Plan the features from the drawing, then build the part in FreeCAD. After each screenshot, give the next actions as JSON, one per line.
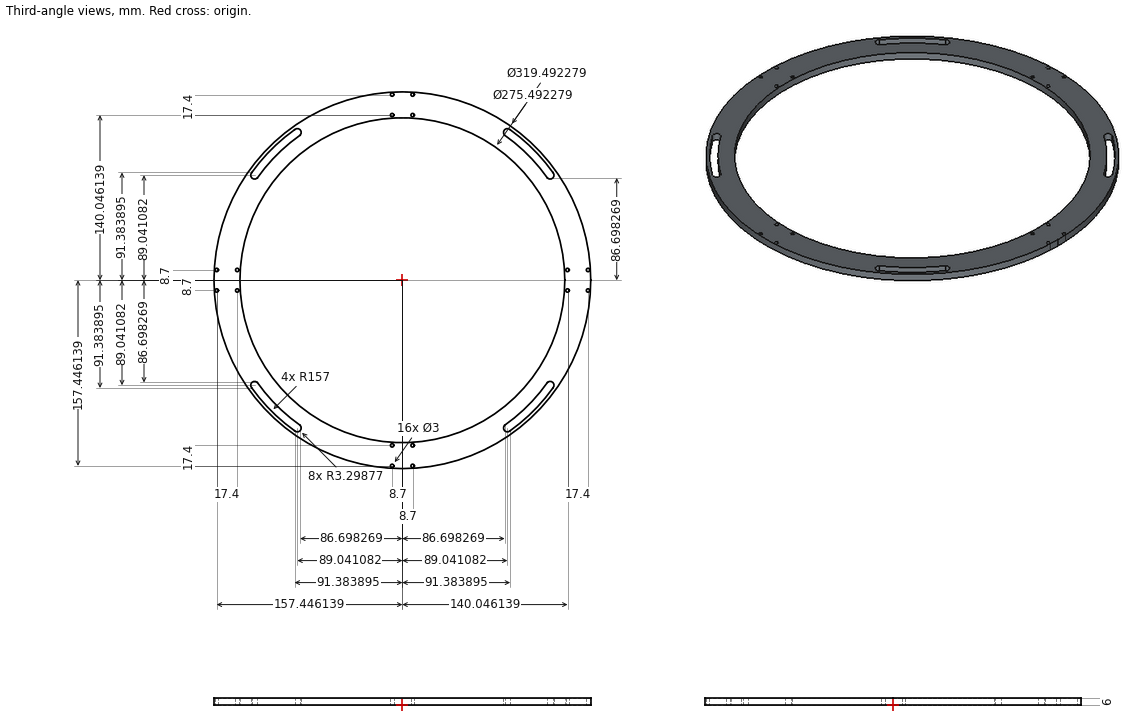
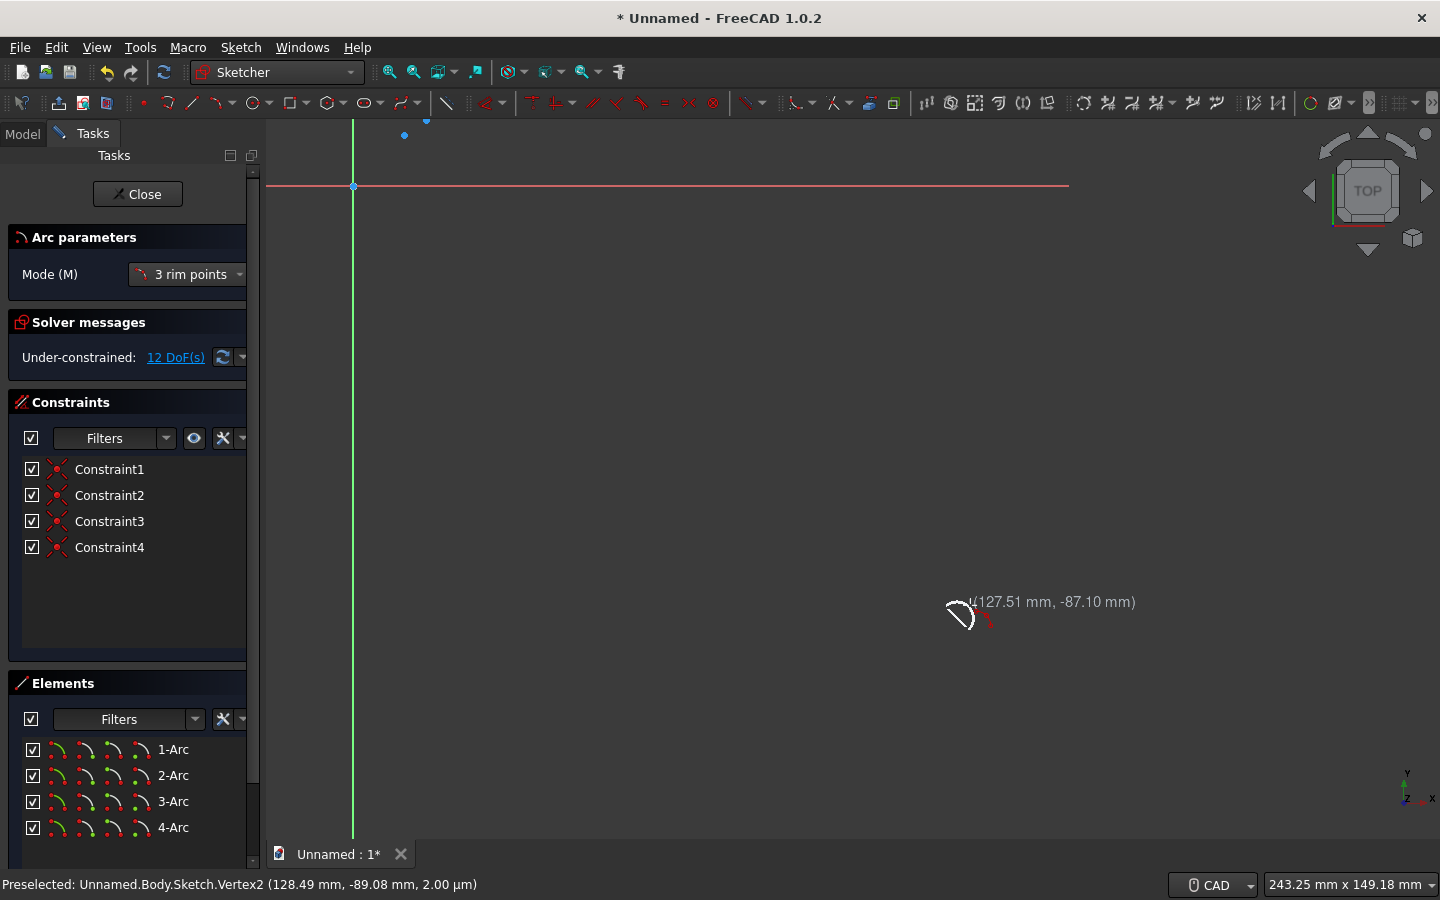
{"action": "left_click", "coordinate": [969, 605]}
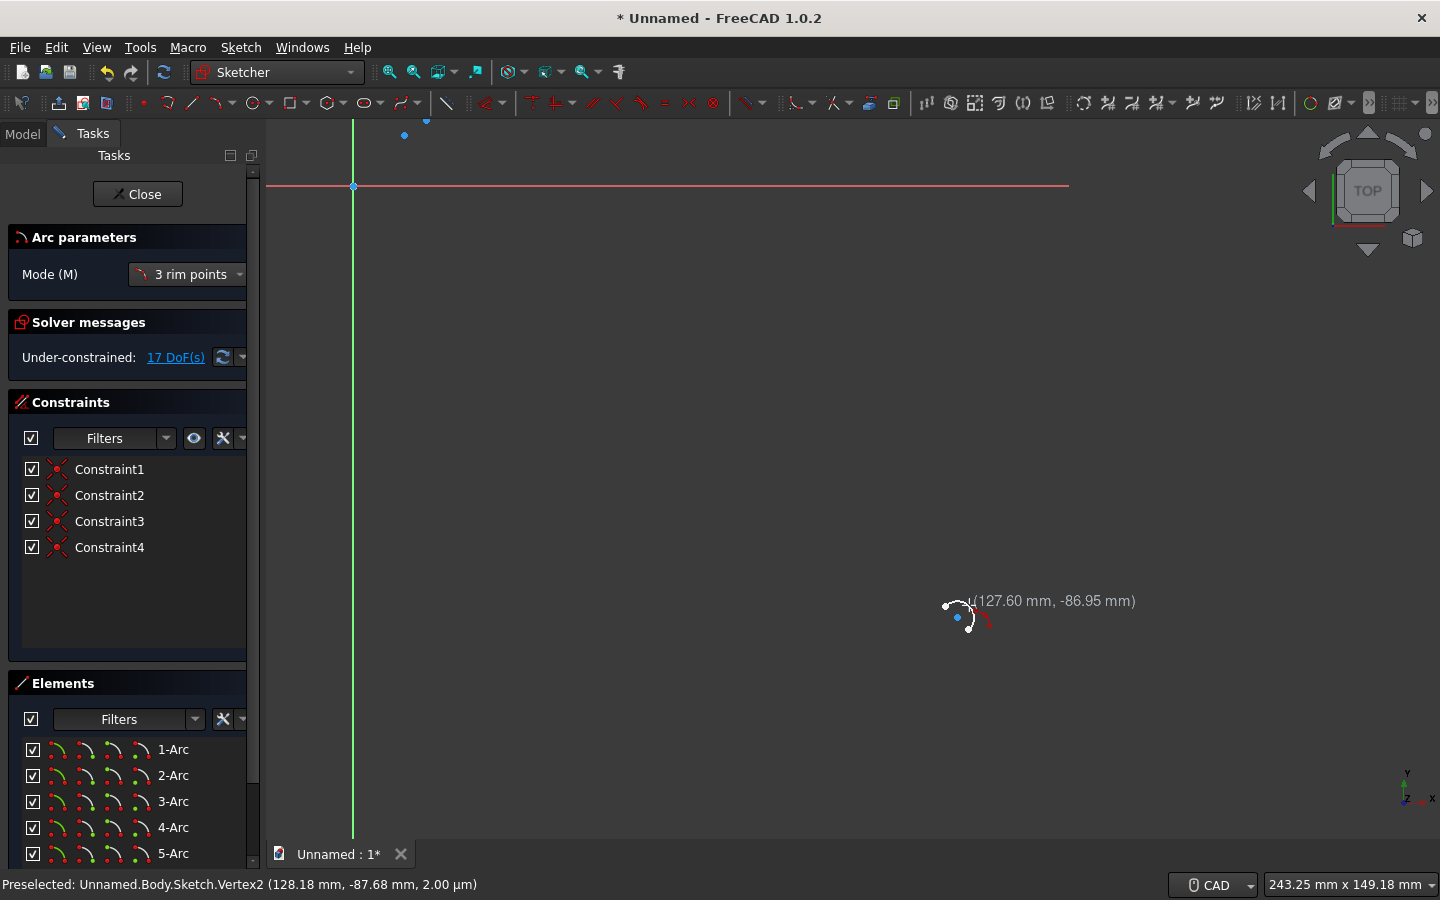
{"action": "left_click", "coordinate": [969, 630]}
{"action": "left_click", "coordinate": [794, 803]}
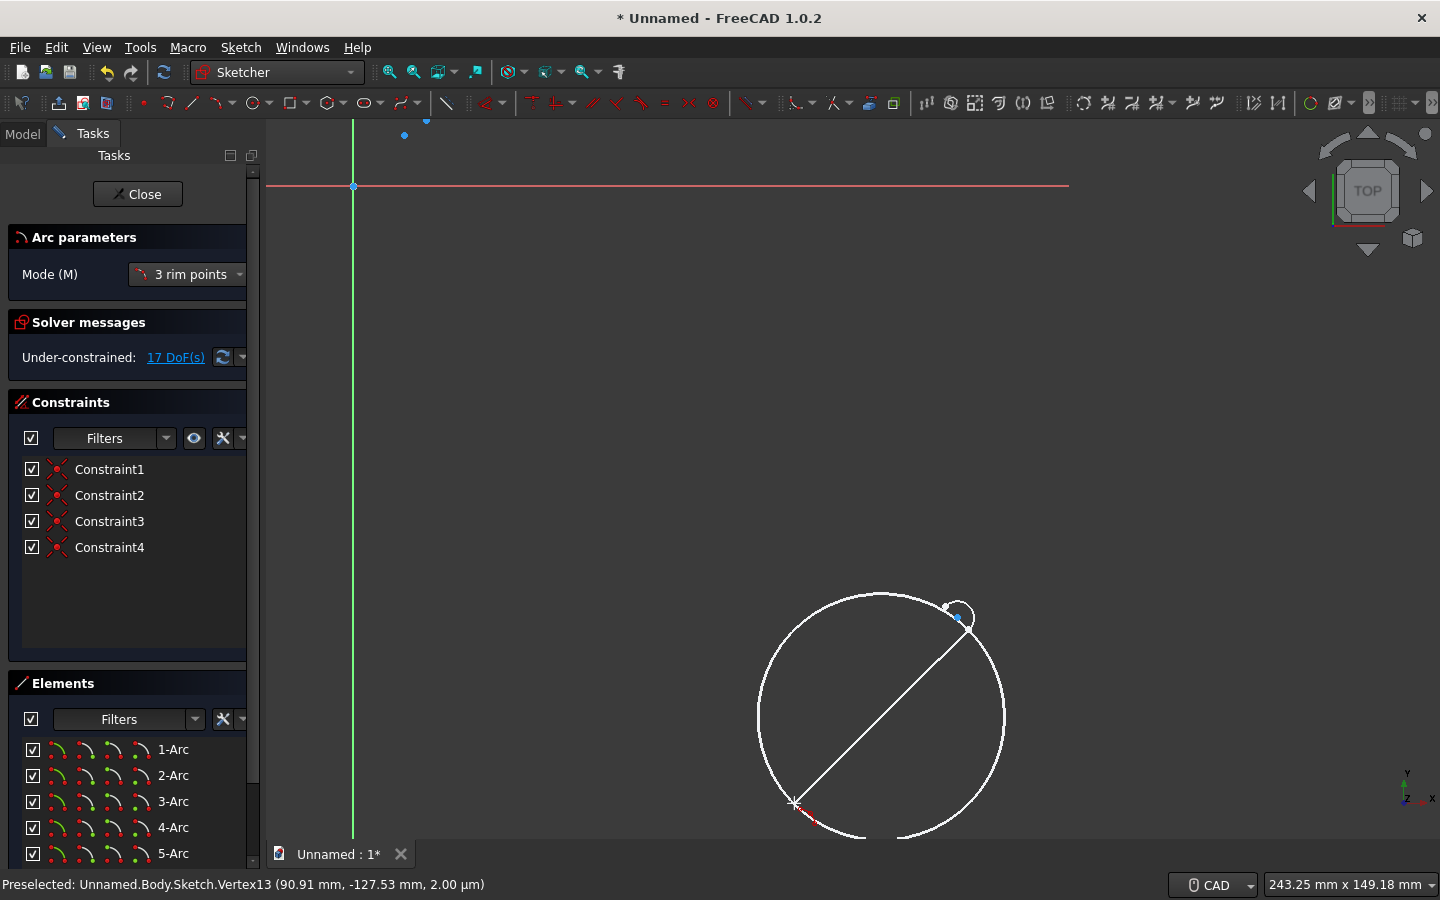
{"action": "scroll", "coordinate": [889, 722], "scroll_direction": "up", "scroll_amount": 3}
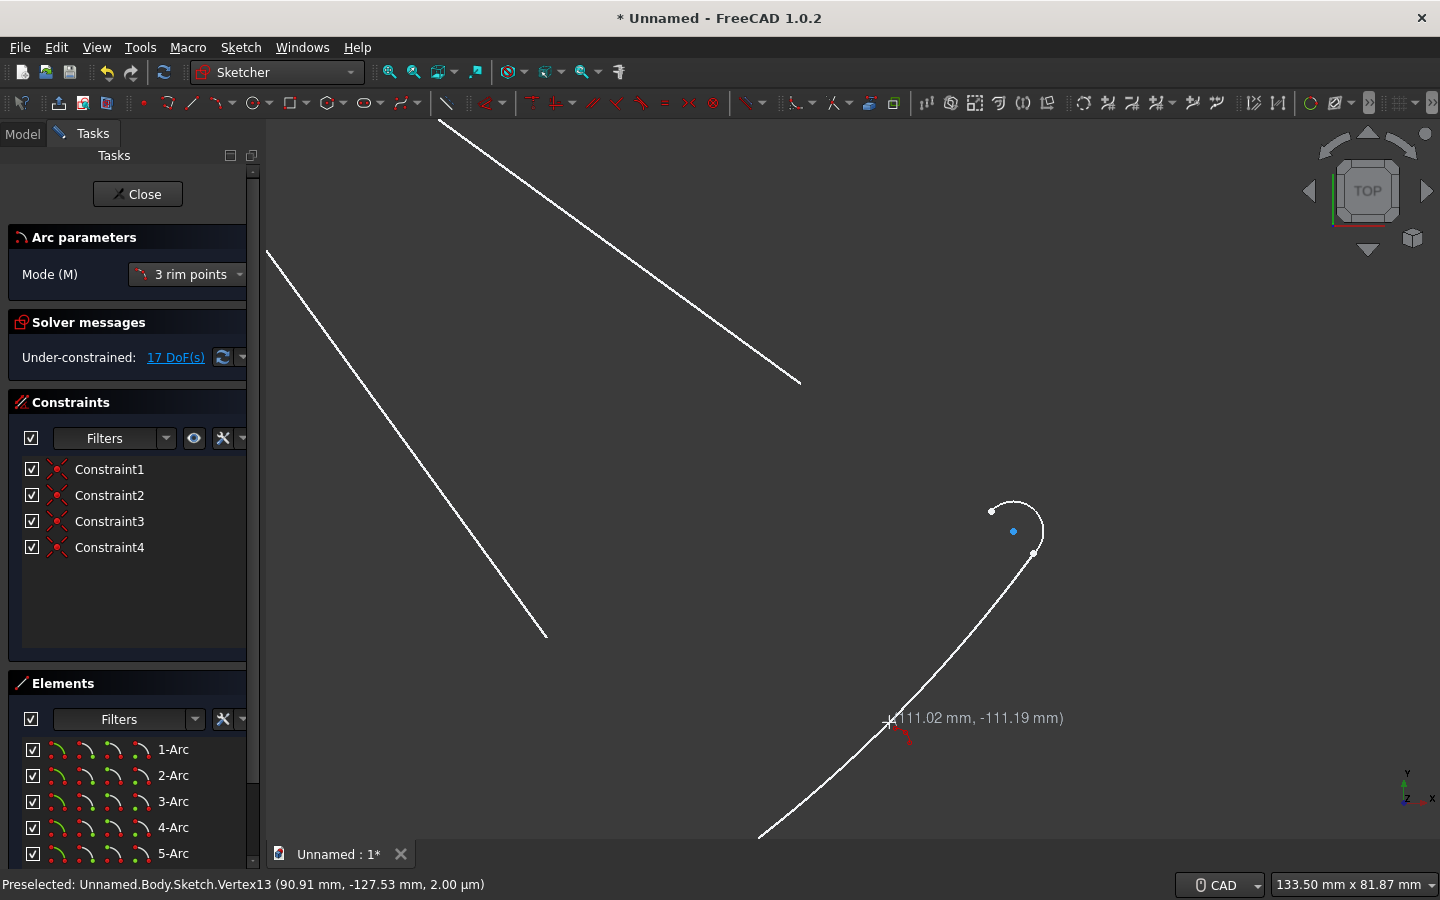
{"action": "left_click", "coordinate": [889, 722]}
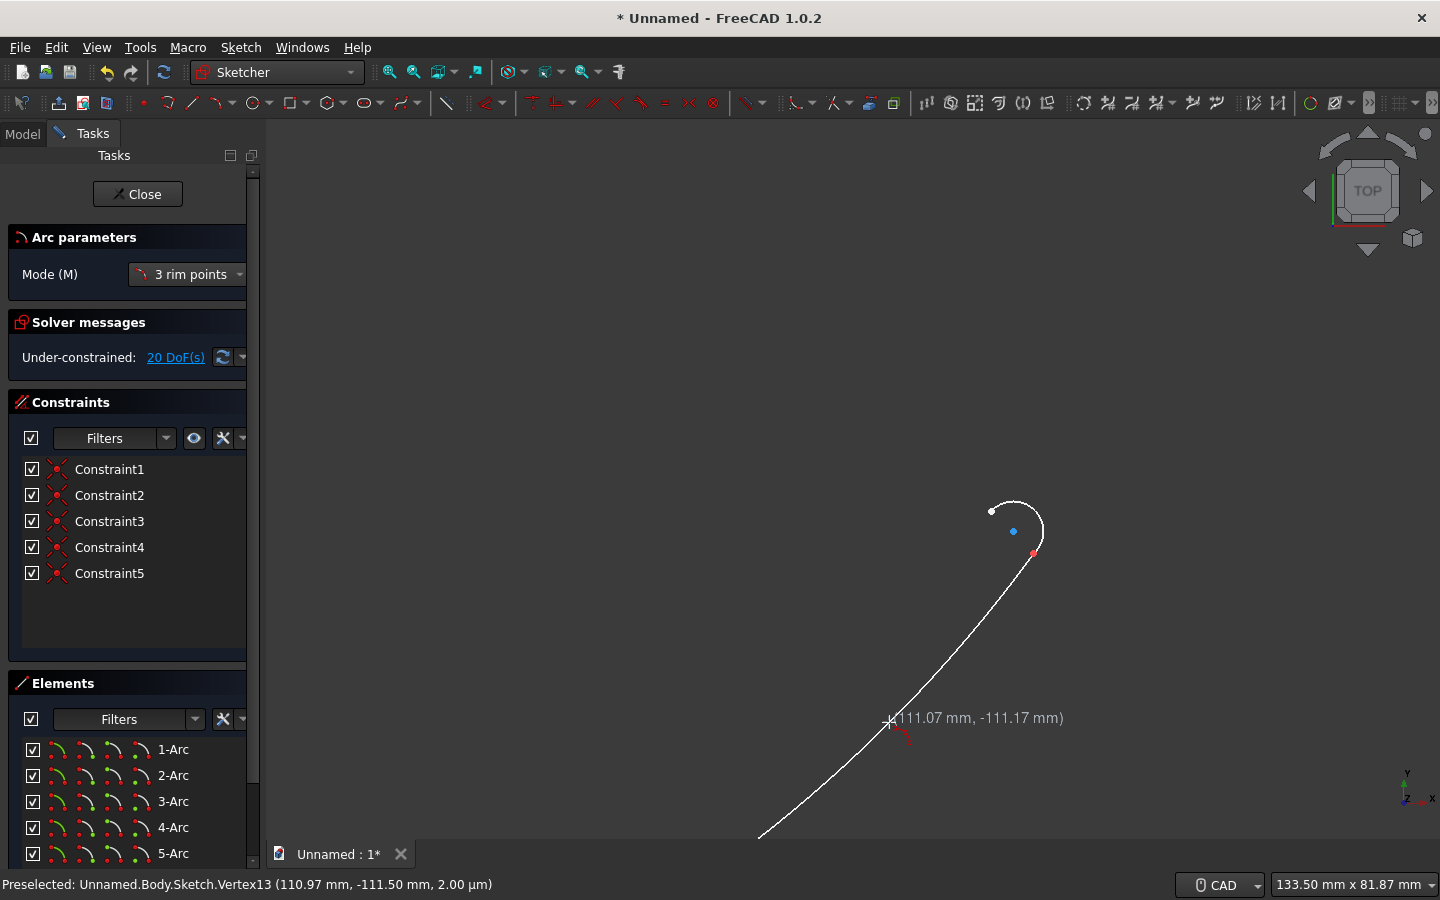
{"action": "scroll", "coordinate": [957, 624], "scroll_direction": "down", "scroll_amount": 9}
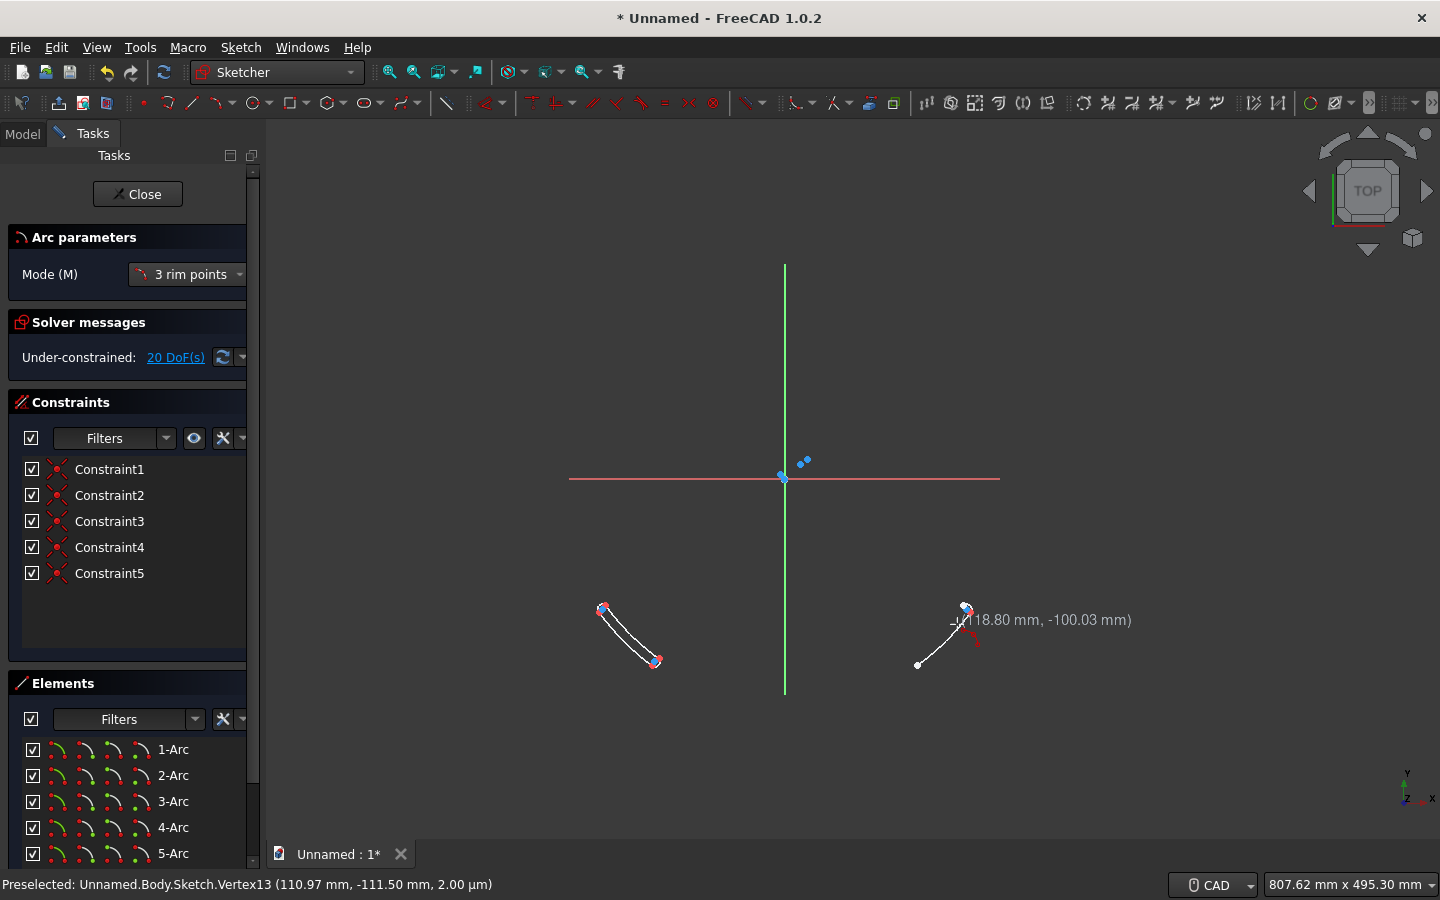
{"action": "left_click", "coordinate": [918, 665]}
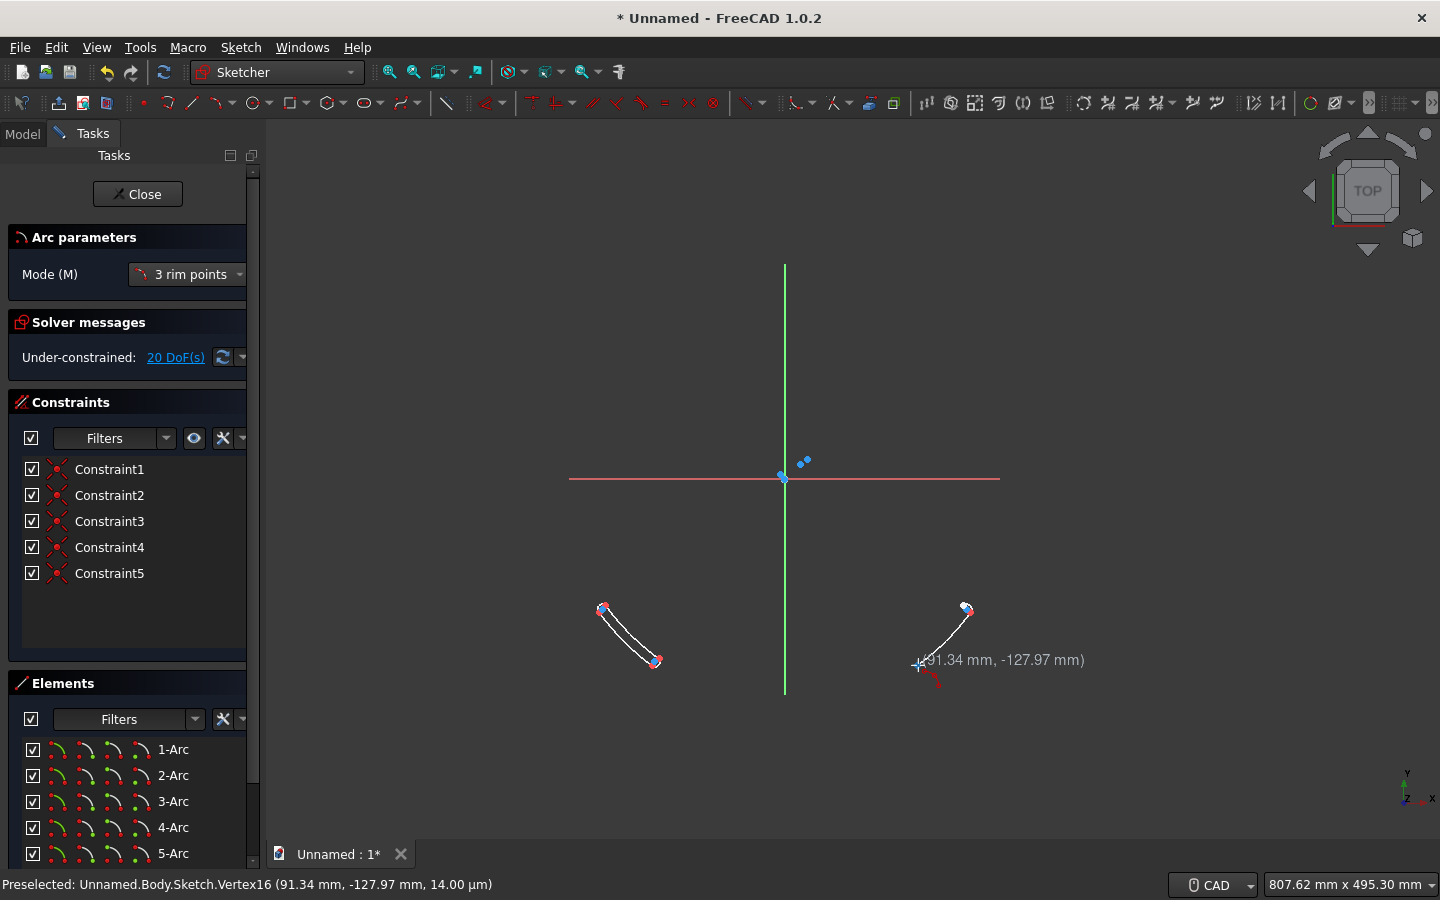
{"action": "scroll", "coordinate": [911, 658], "scroll_direction": "up", "scroll_amount": 3}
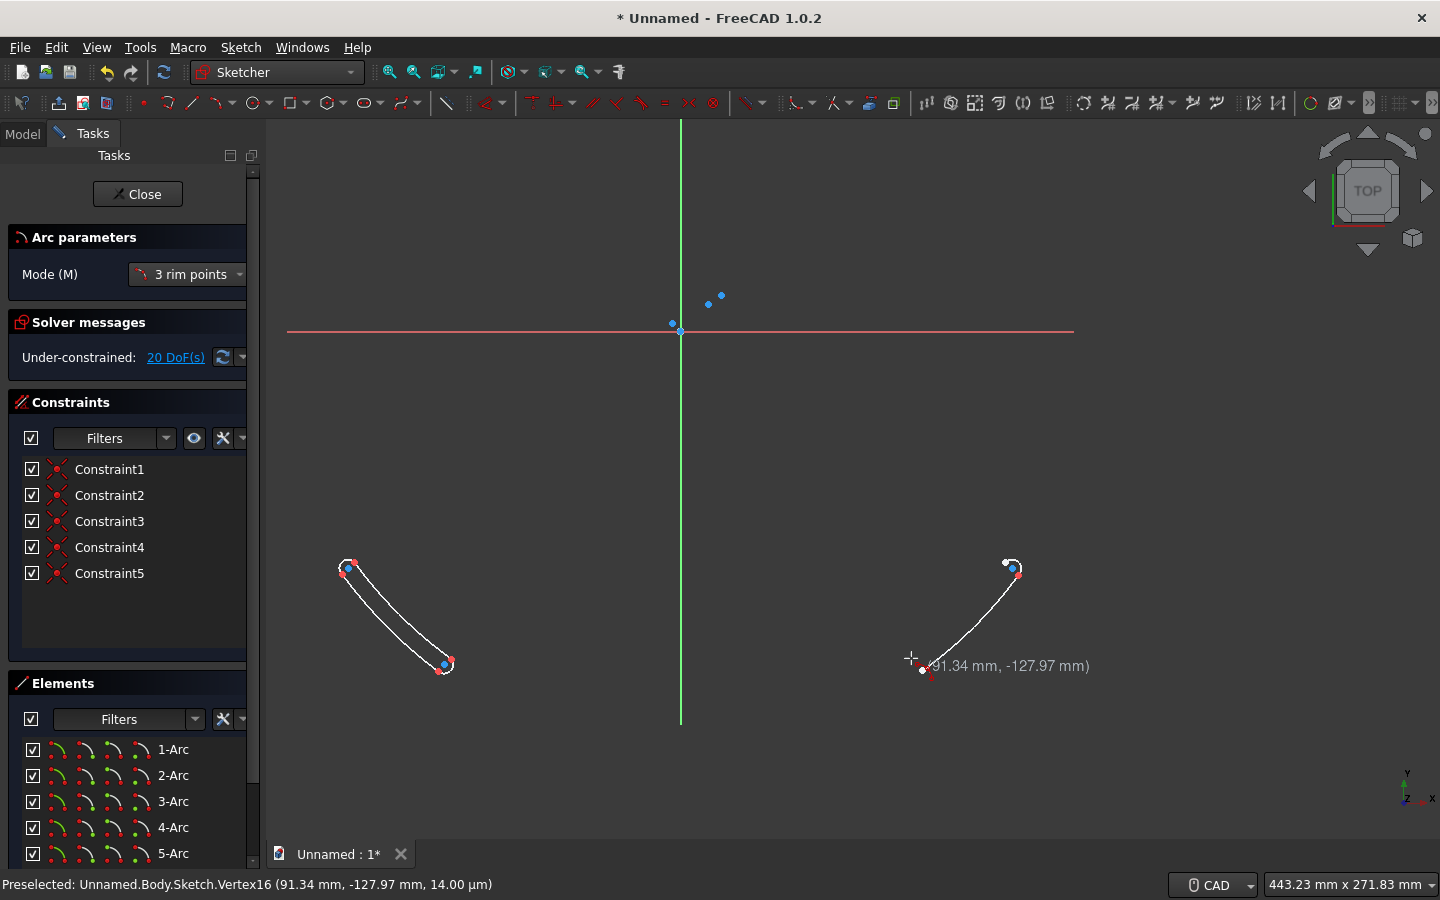
{"action": "left_click", "coordinate": [910, 658]}